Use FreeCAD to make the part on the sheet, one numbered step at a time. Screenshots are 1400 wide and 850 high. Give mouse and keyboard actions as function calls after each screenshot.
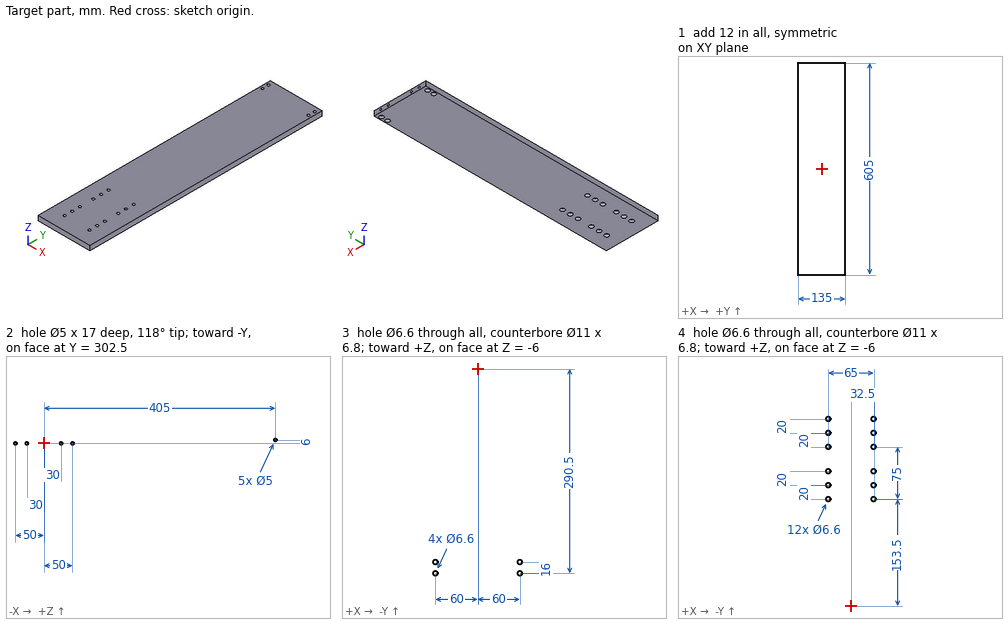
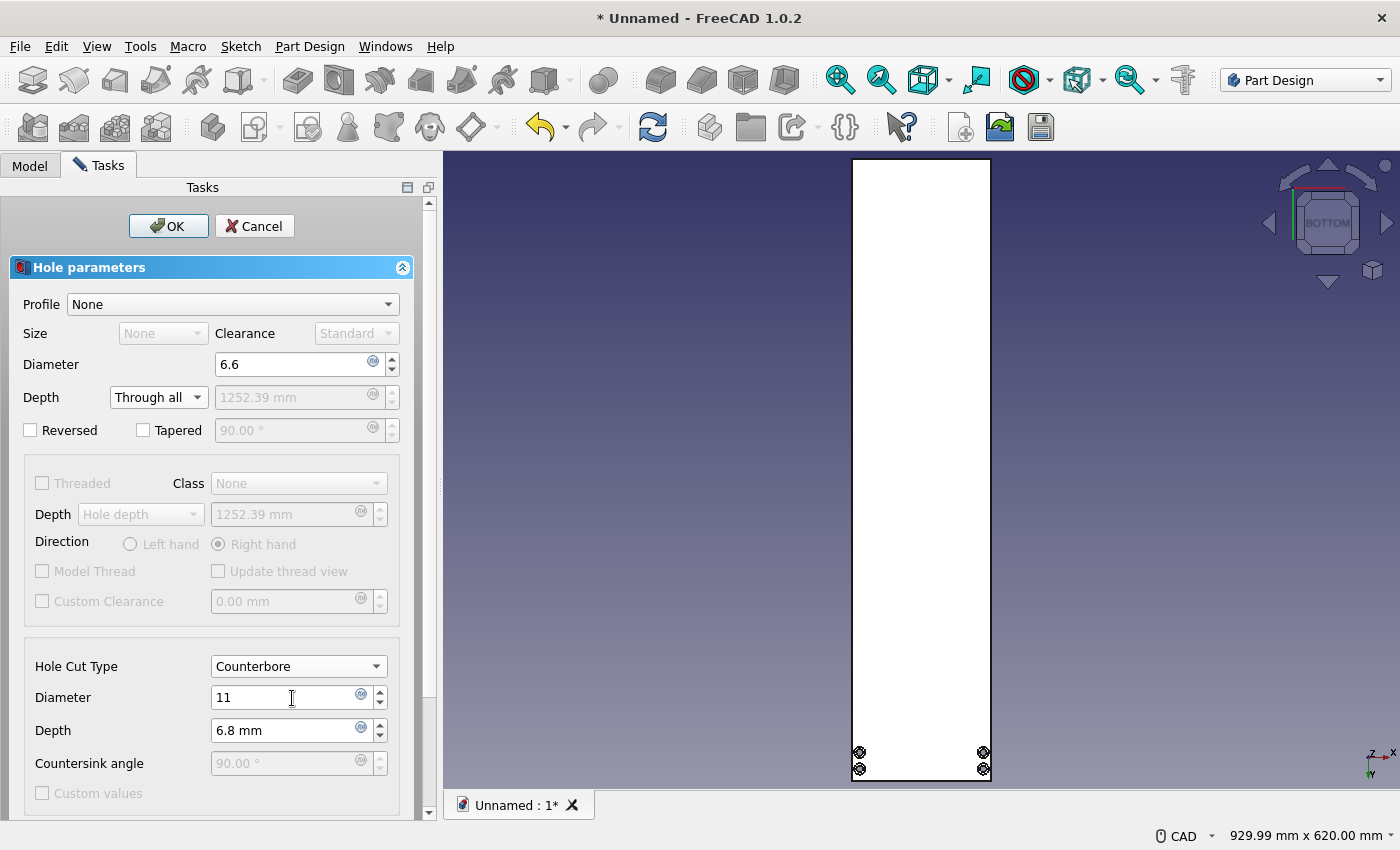
click(169, 226)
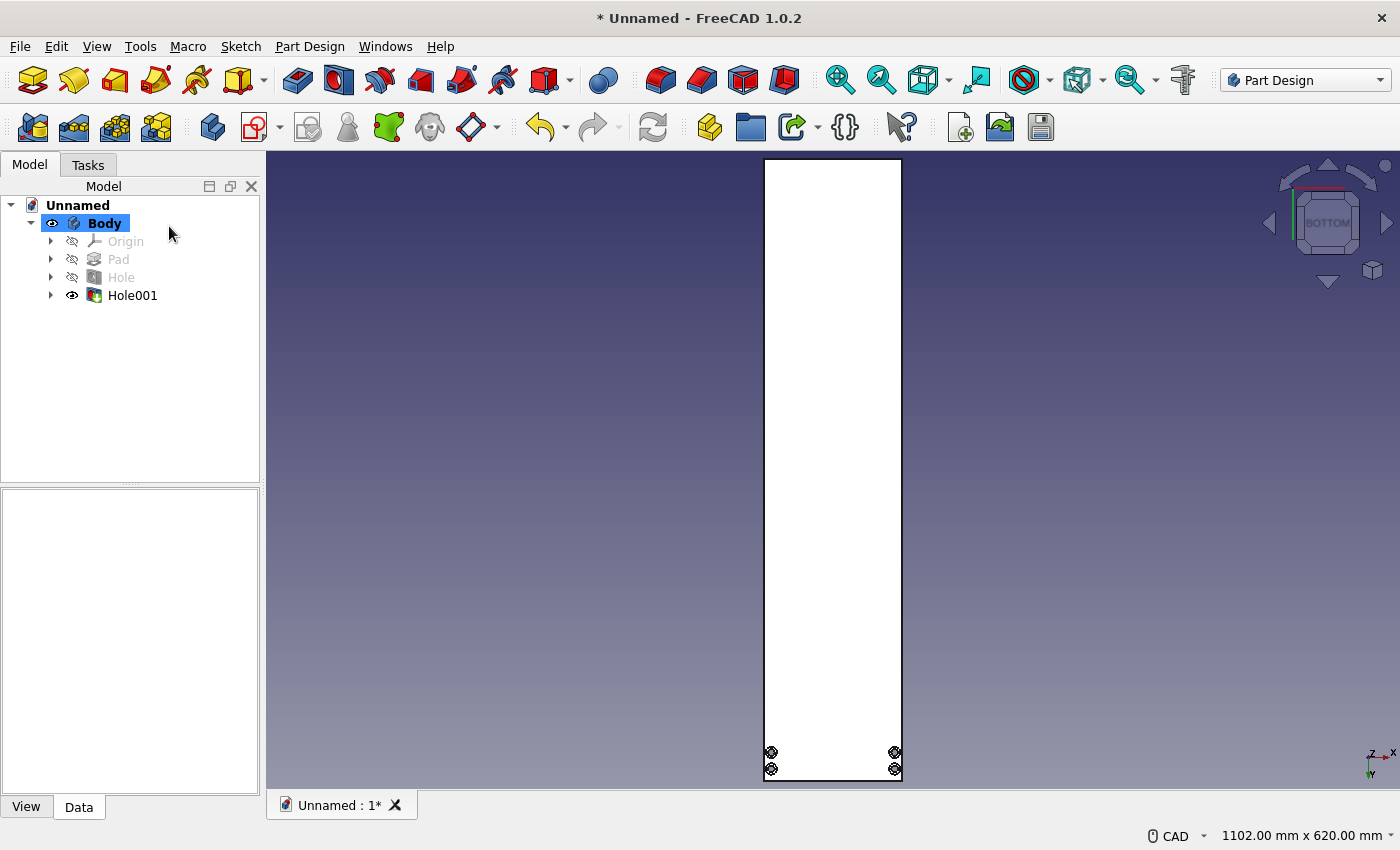
click(833, 647)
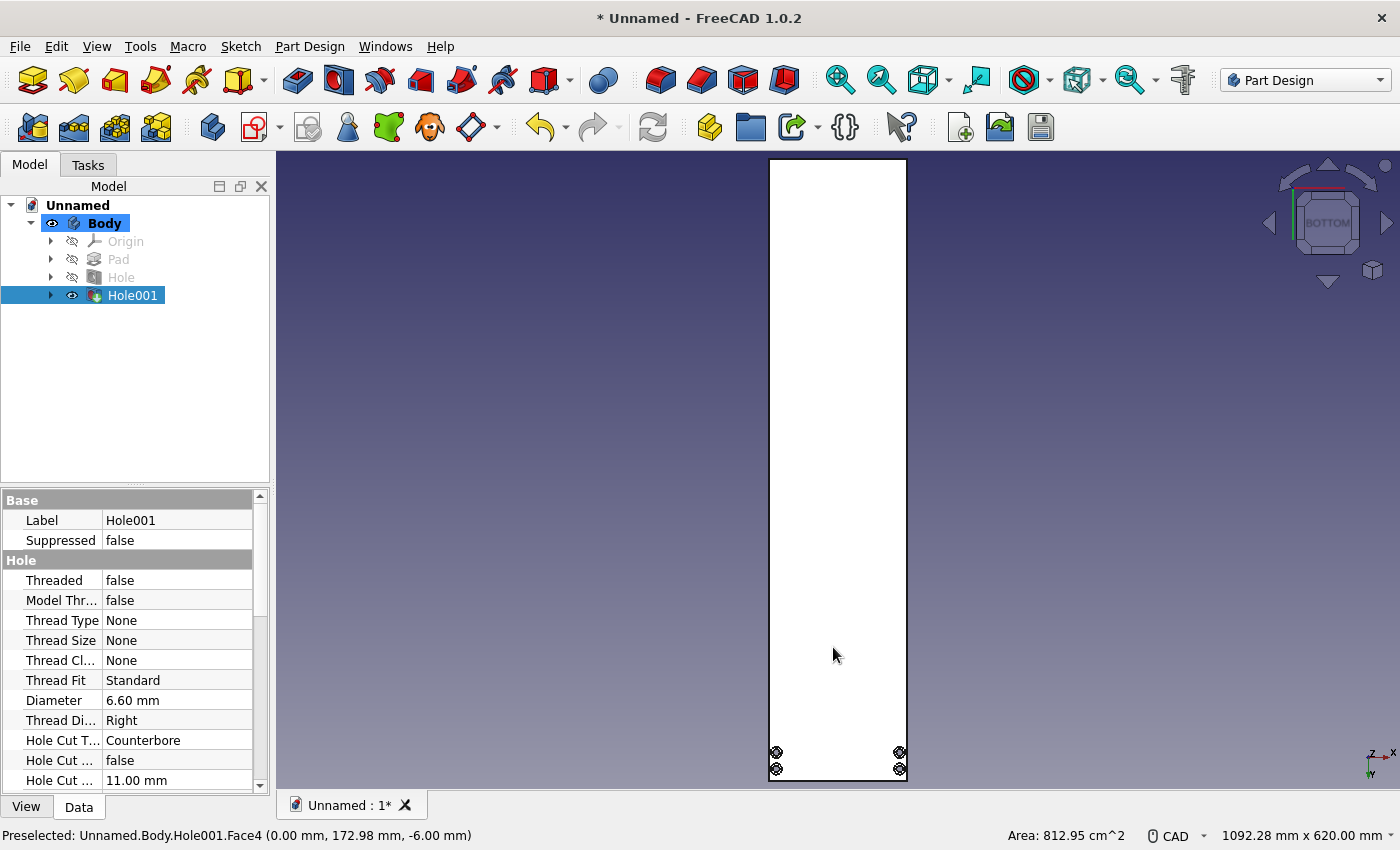
click(254, 128)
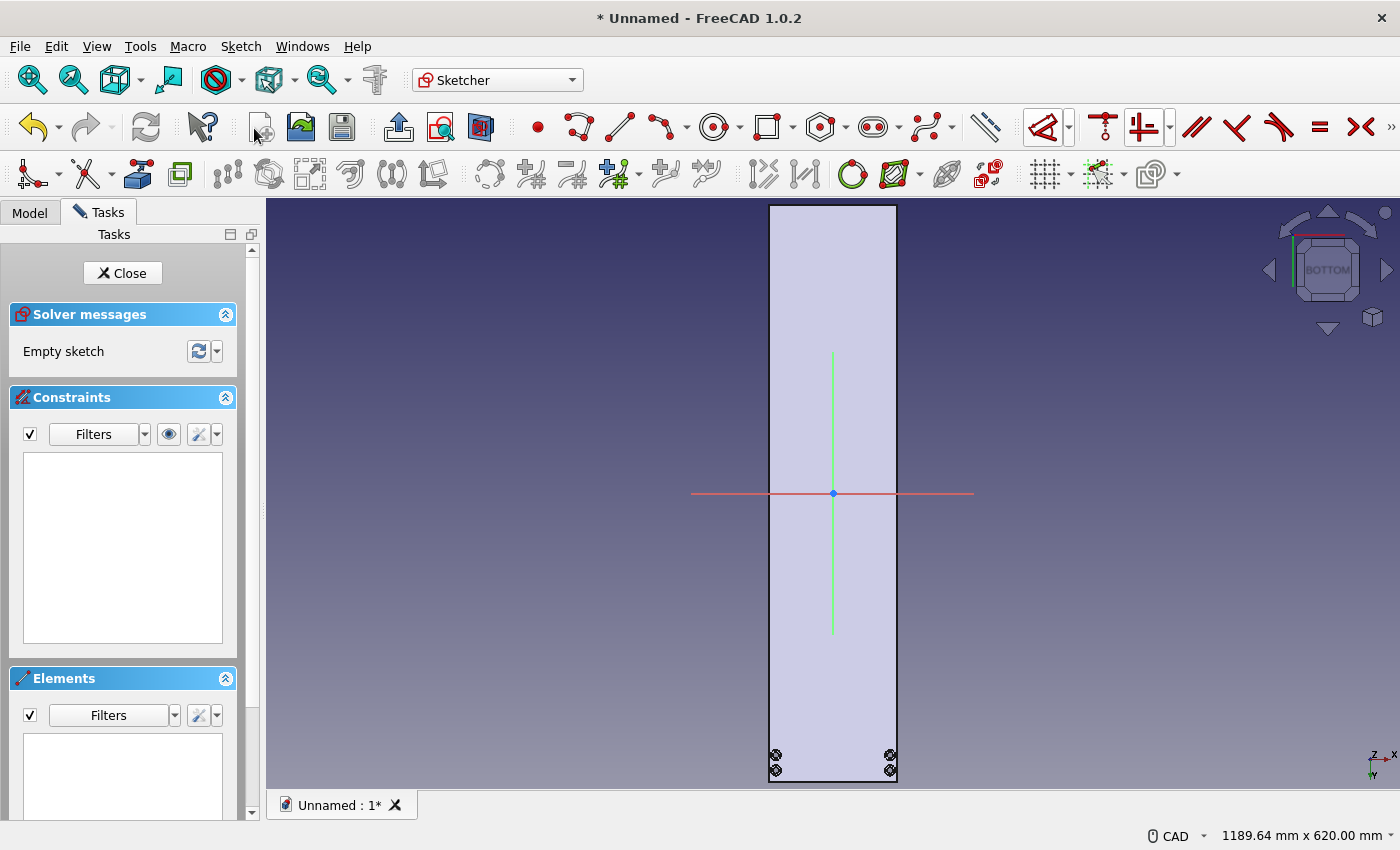
scroll(455, 761, down, 1)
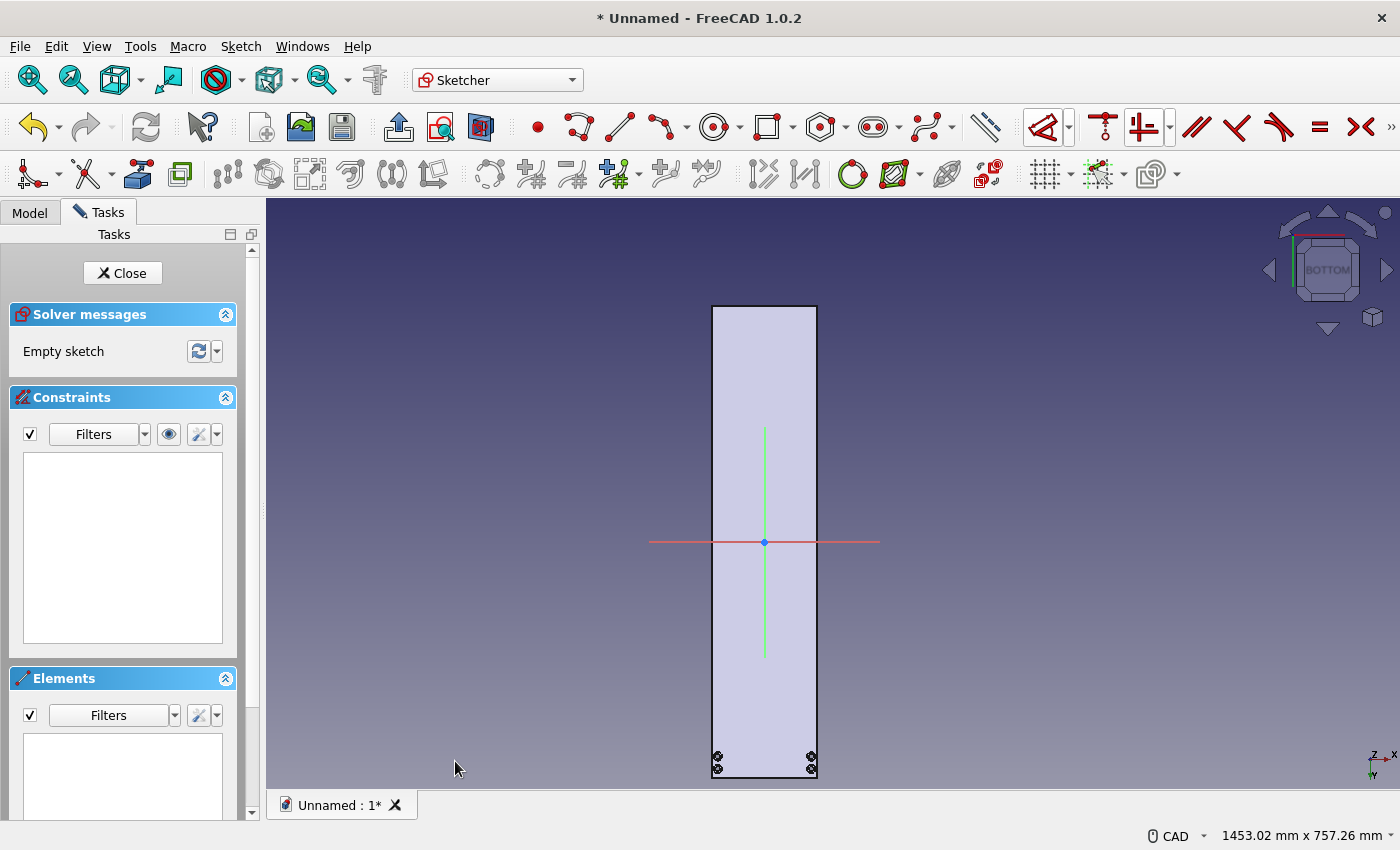
scroll(765, 366, up, 3)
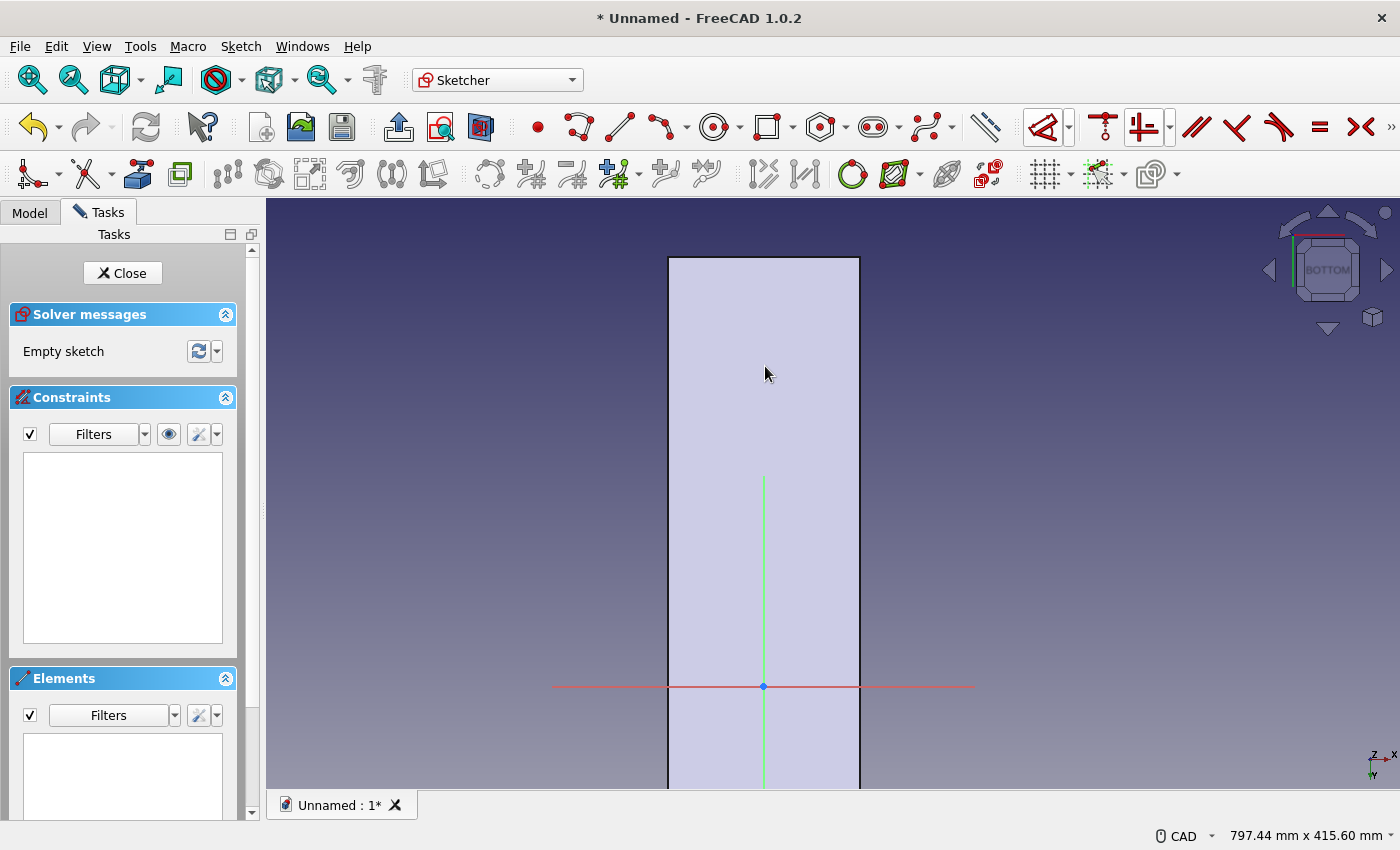
click(714, 128)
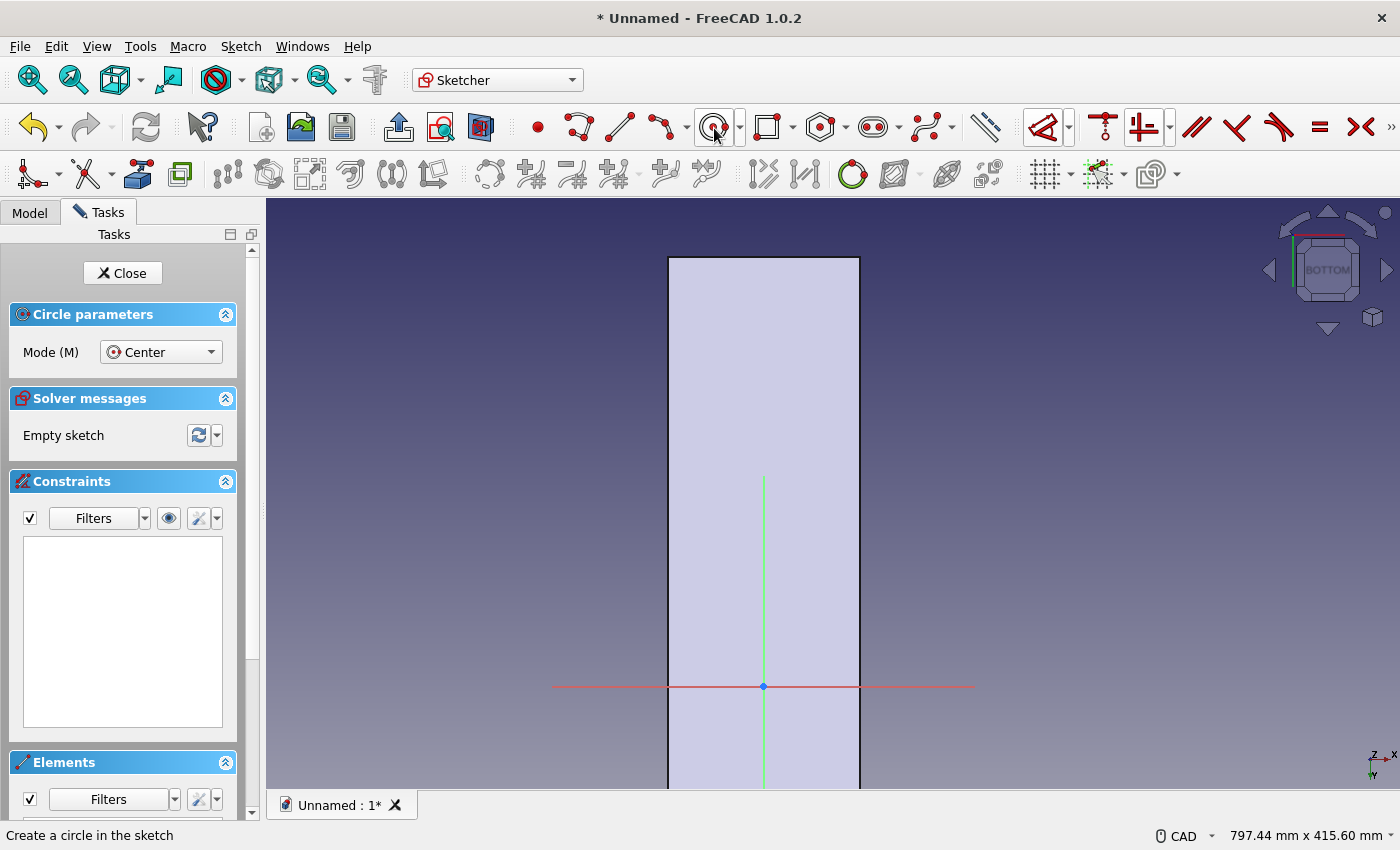
scroll(810, 468, up, 8)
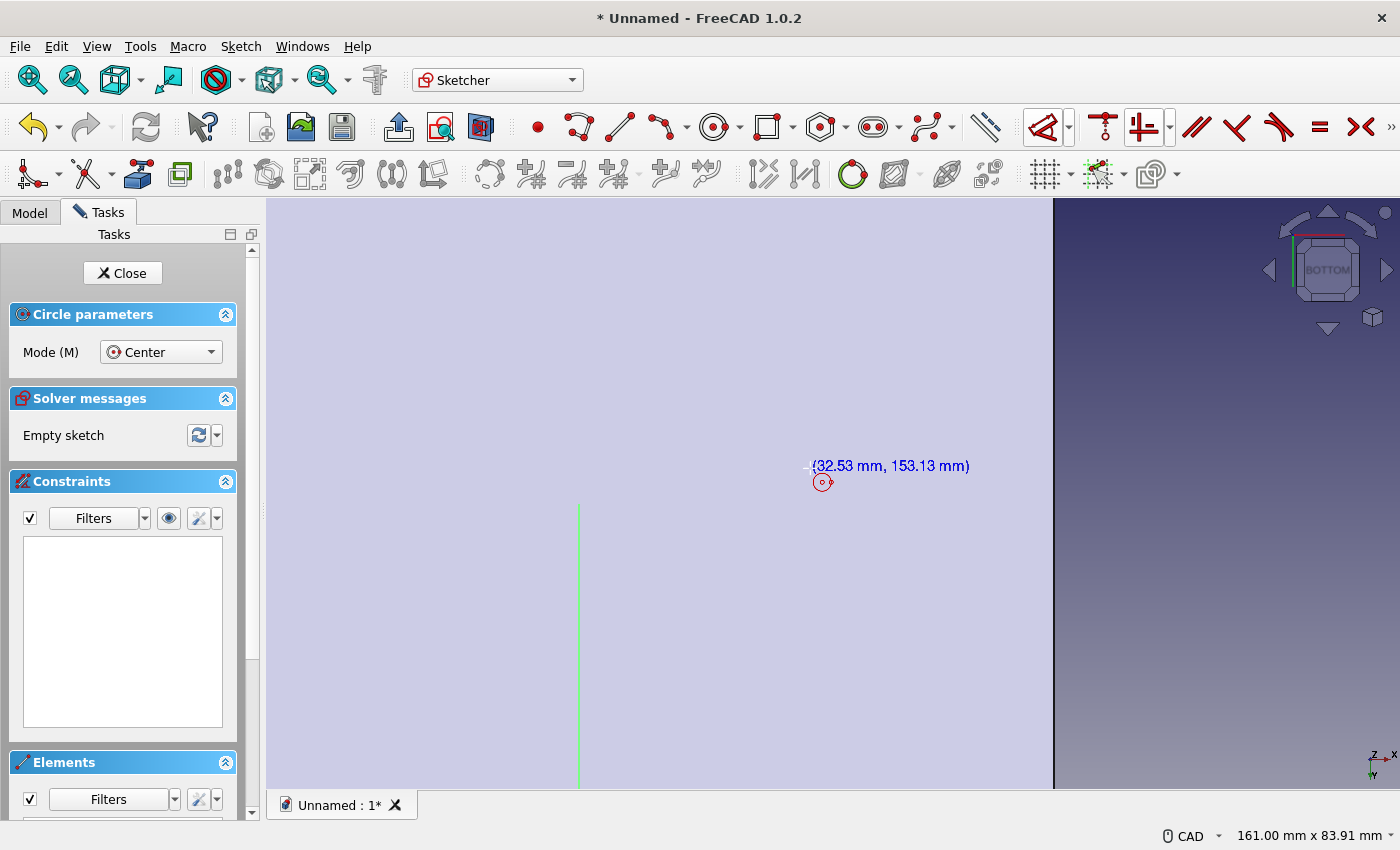
scroll(811, 468, down, 8)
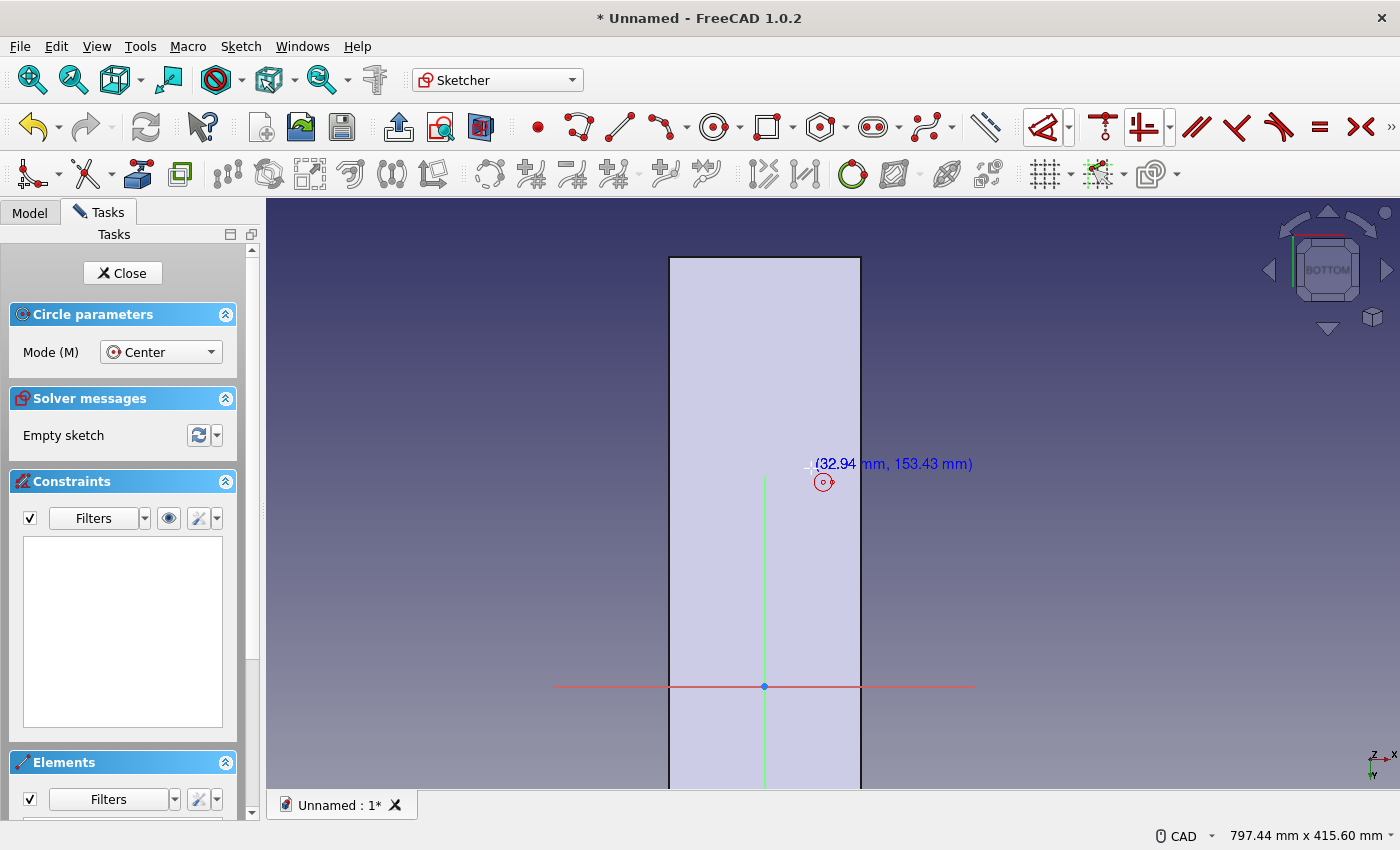
click(811, 468)
move(814, 465)